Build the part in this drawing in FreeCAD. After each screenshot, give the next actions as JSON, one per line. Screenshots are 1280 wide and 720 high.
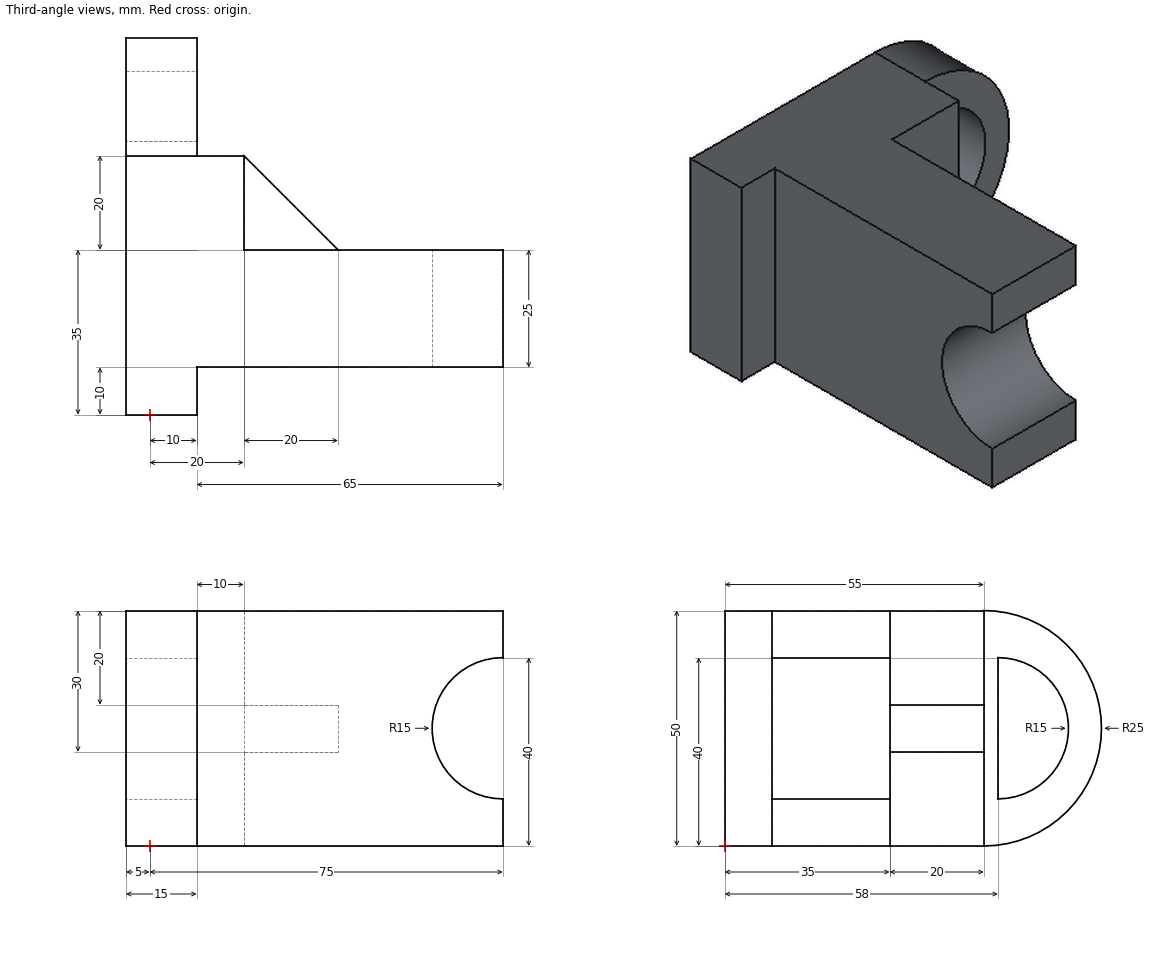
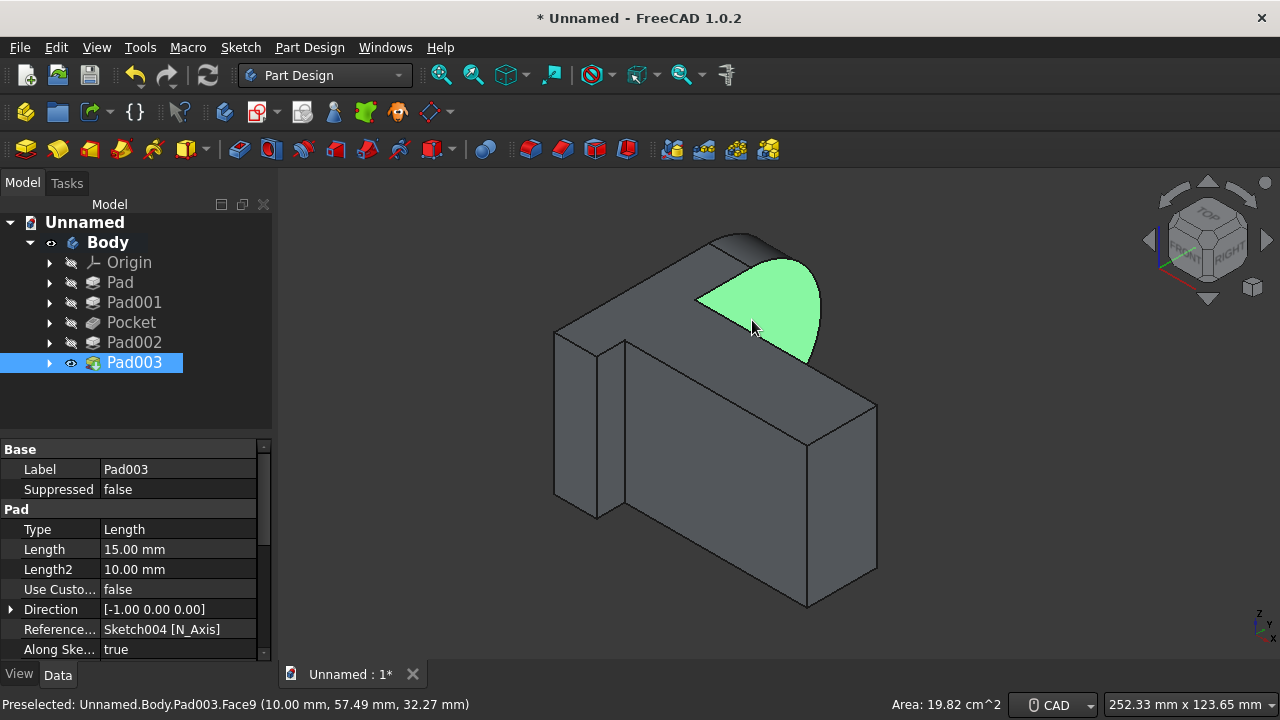
{"action": "left_click", "coordinate": [258, 112]}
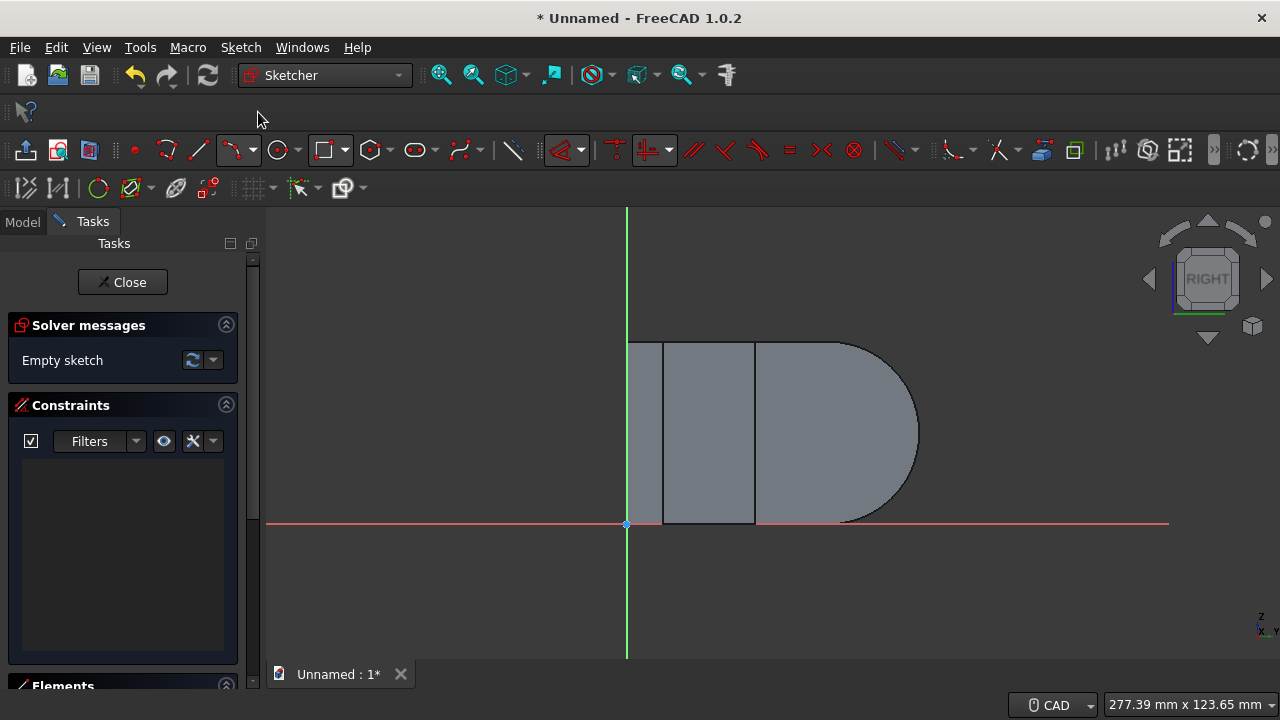
{"action": "scroll", "coordinate": [774, 433], "scroll_direction": "up", "scroll_amount": 2}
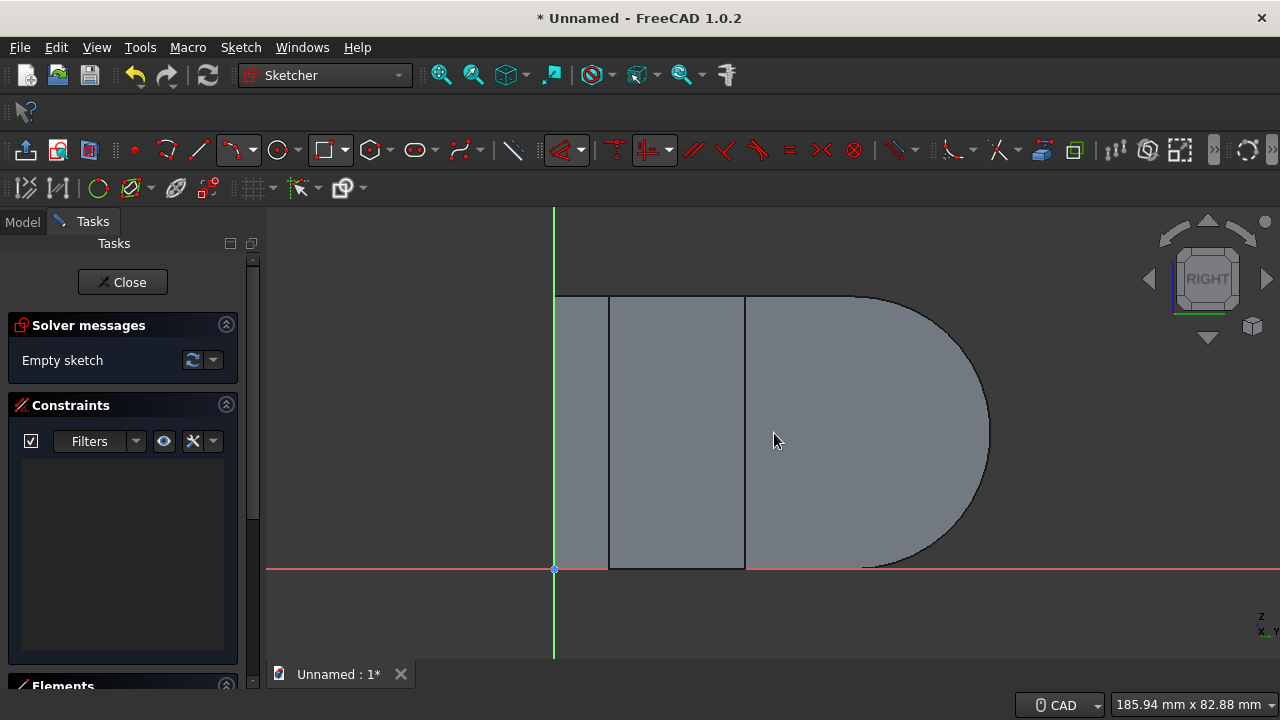
{"action": "key", "text": "g r"}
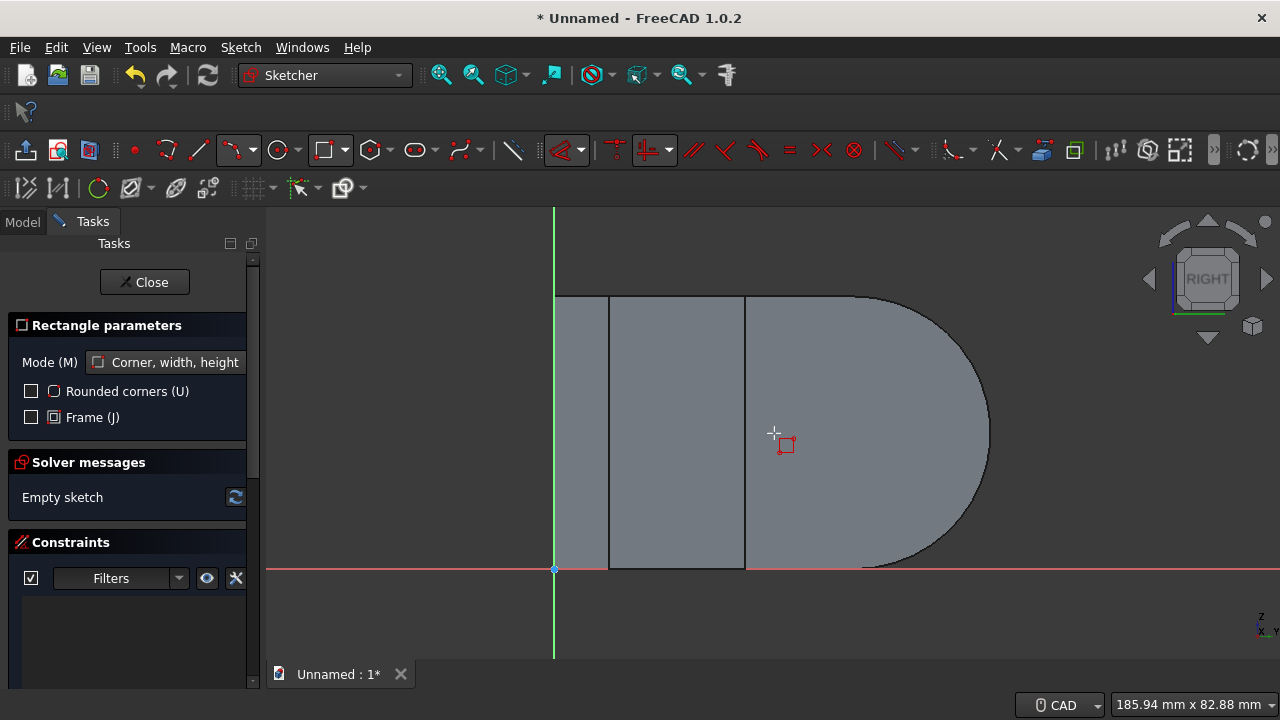
{"action": "left_click", "coordinate": [745, 296]}
{"action": "left_click", "coordinate": [854, 569]}
{"action": "key", "text": "Escape"}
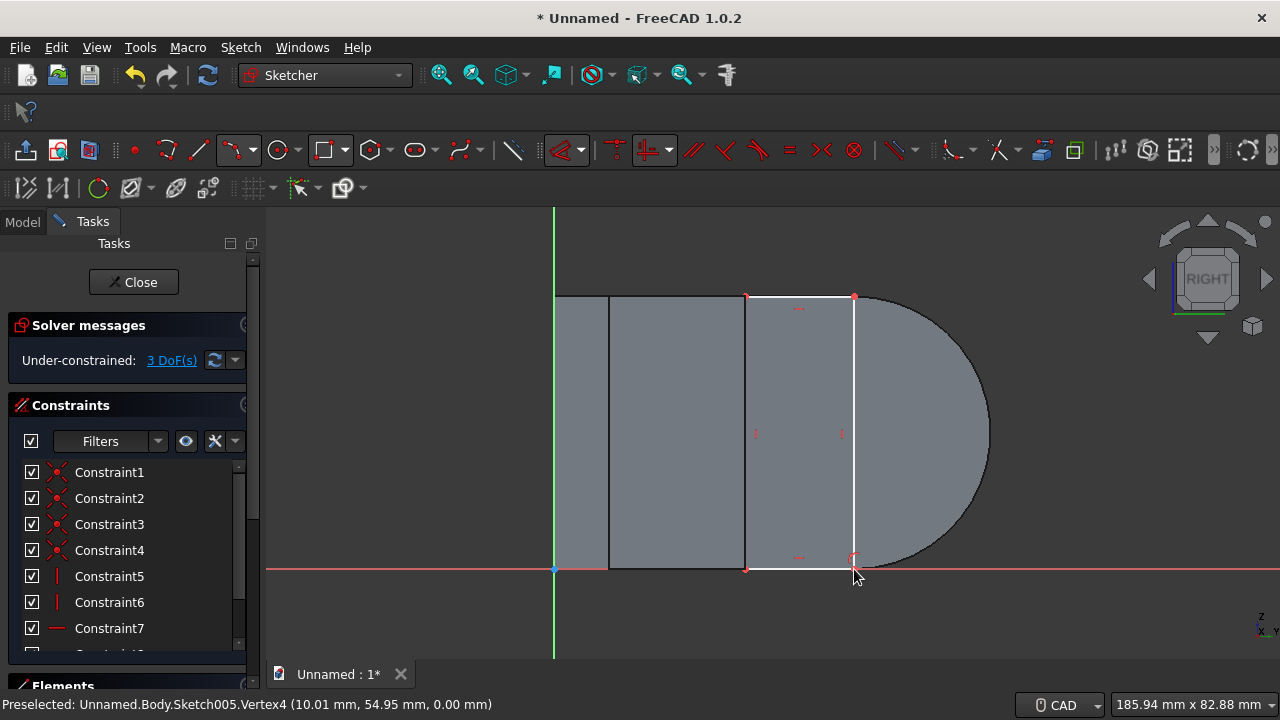
{"action": "left_click", "coordinate": [745, 379]}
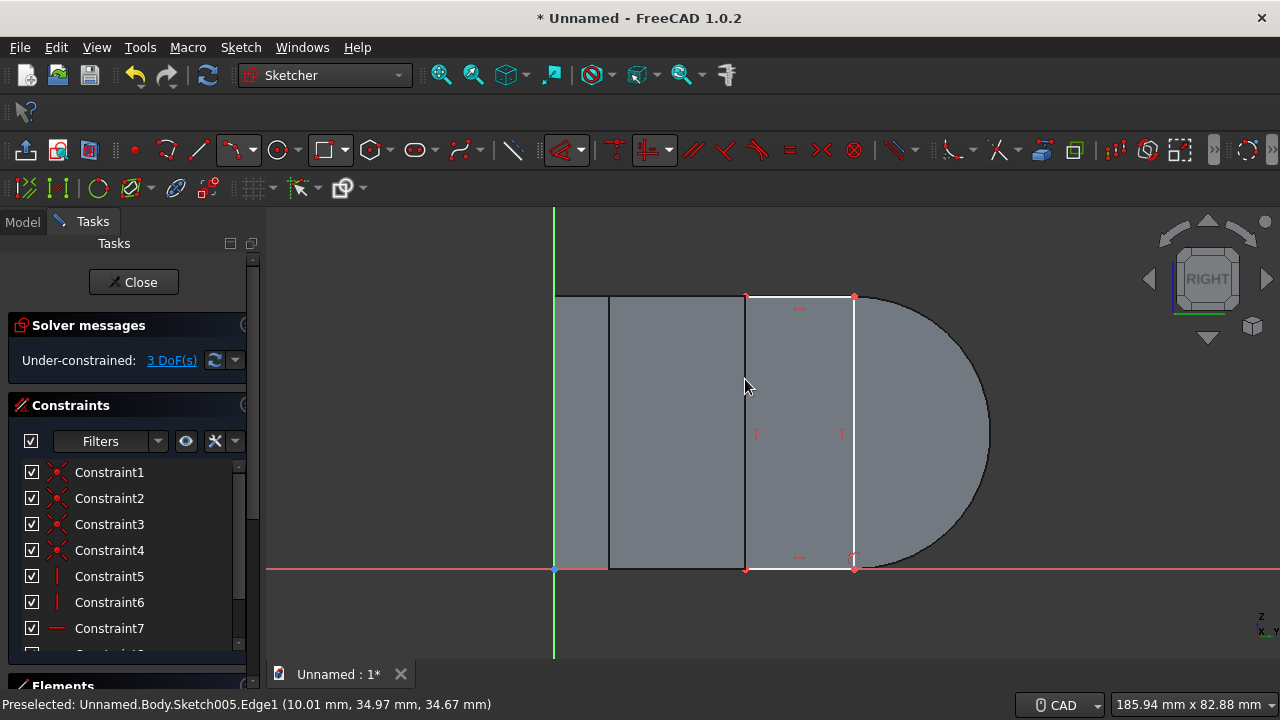
{"action": "left_click", "coordinate": [584, 150]}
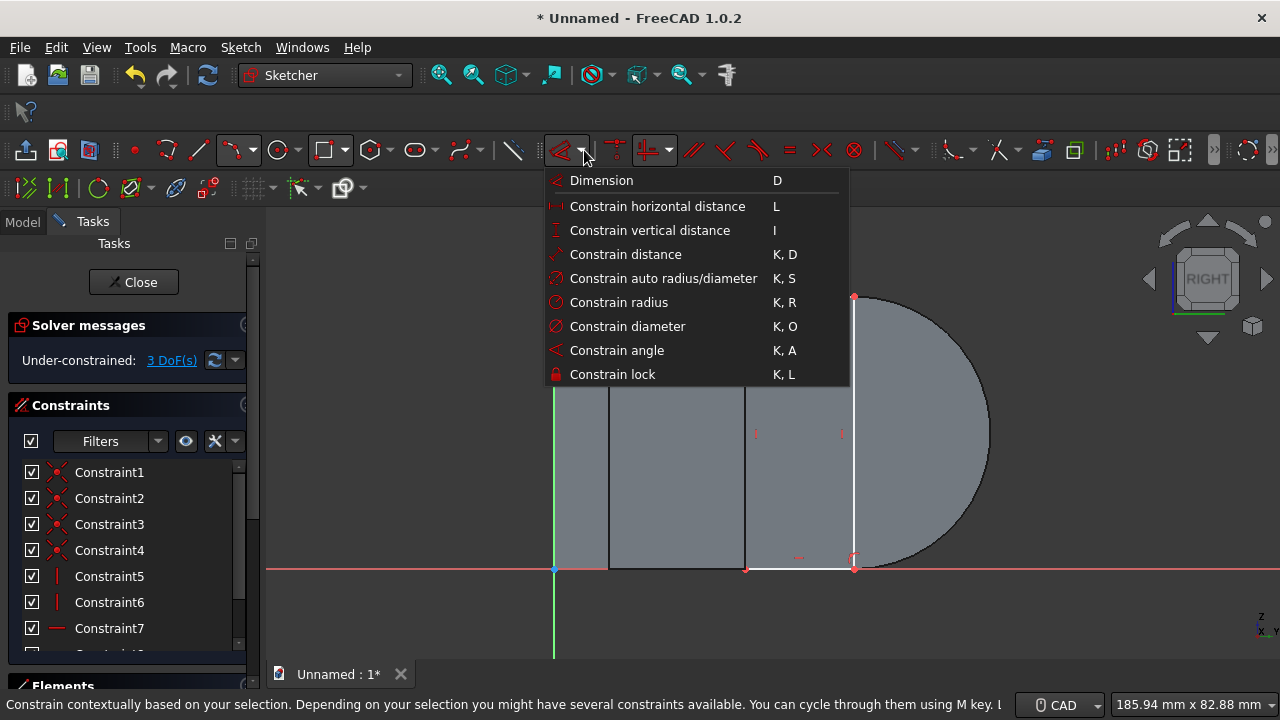
{"action": "left_click", "coordinate": [697, 230]}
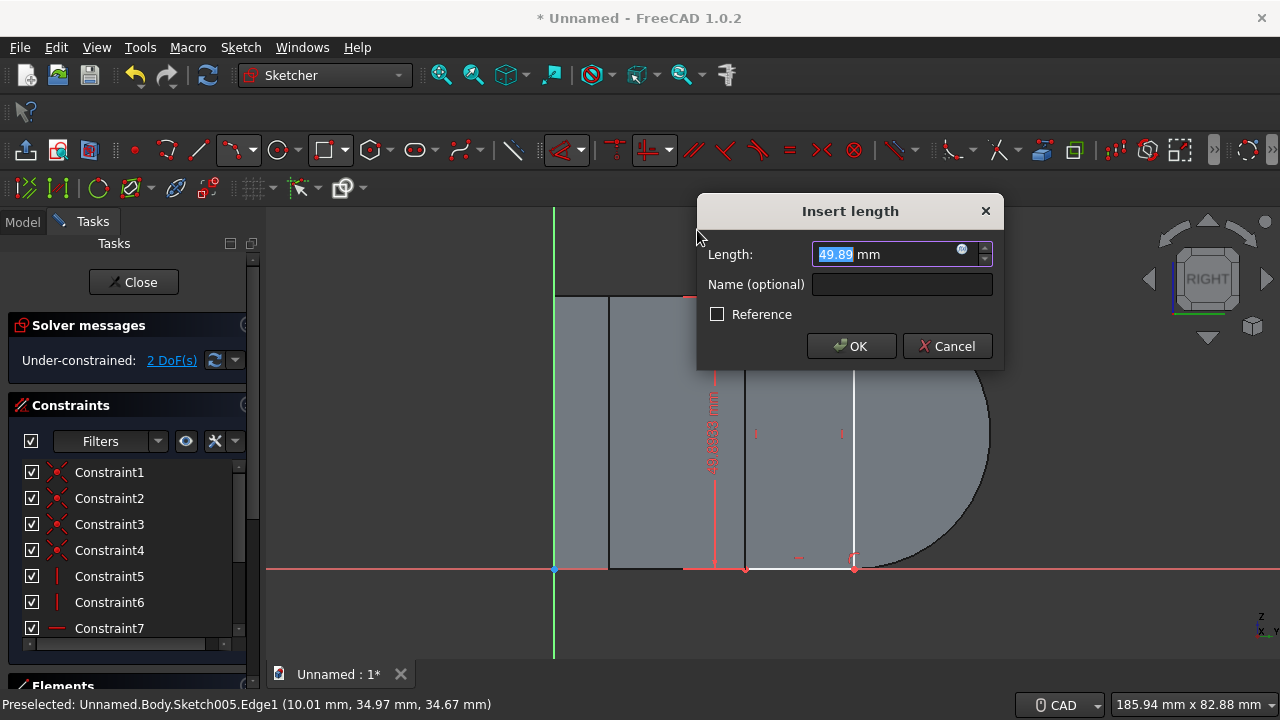
{"action": "type", "text": "50"}
{"action": "key", "text": "Return"}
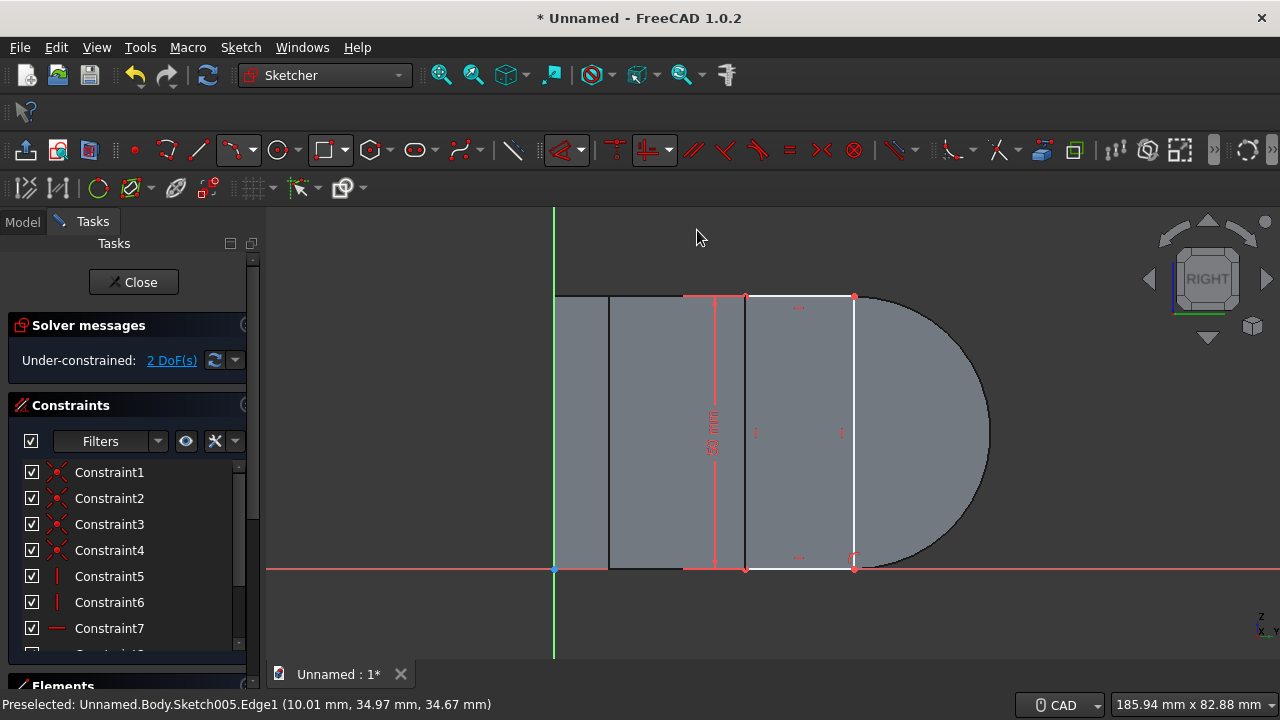
{"action": "left_click", "coordinate": [778, 569]}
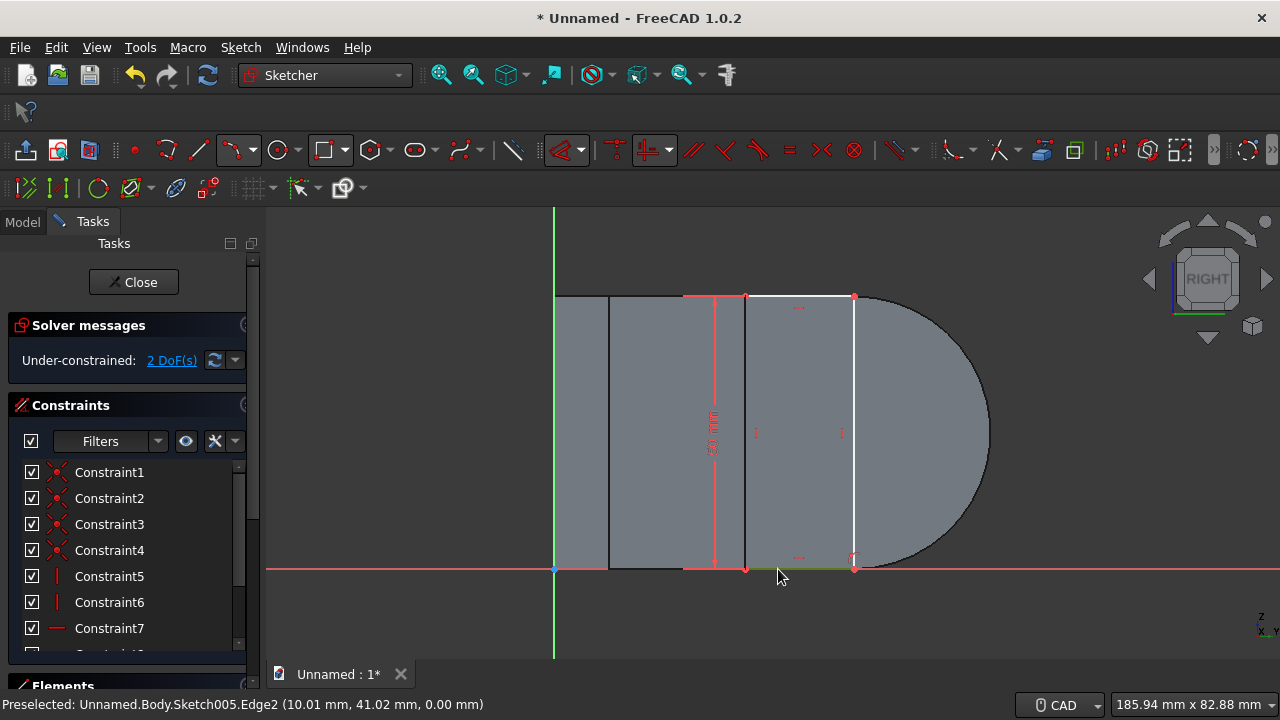
{"action": "key", "text": "l"}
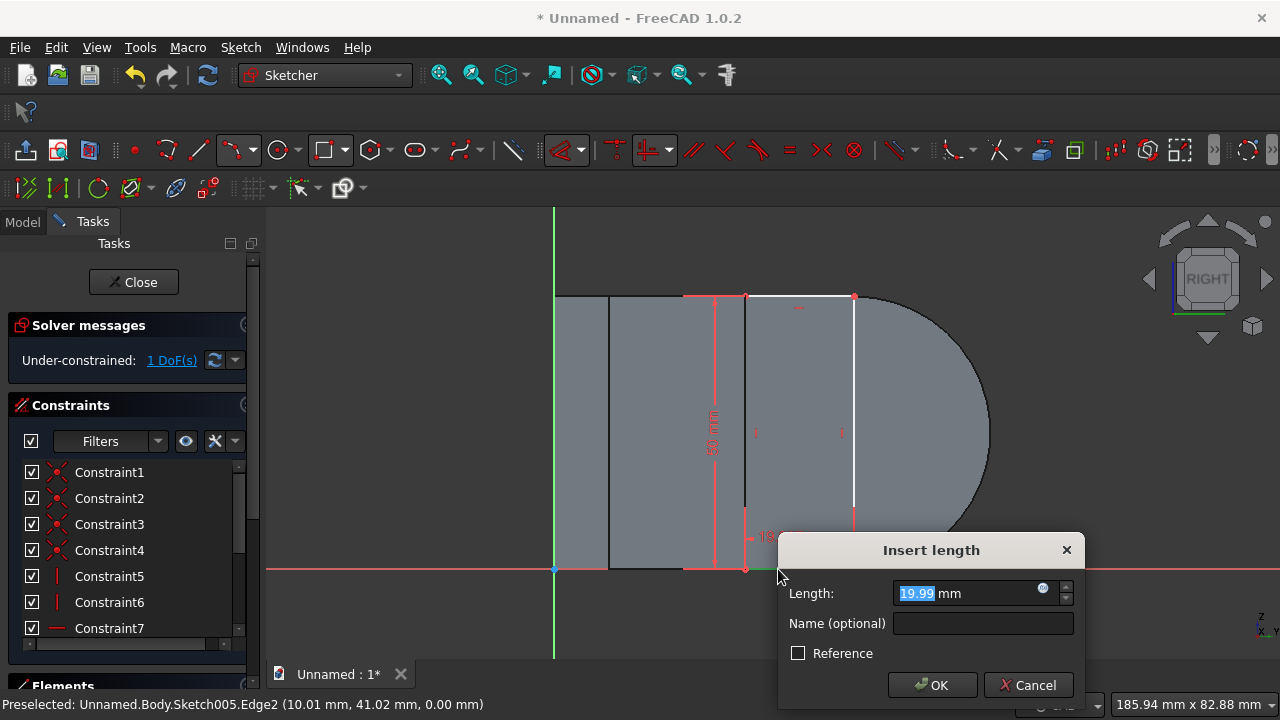
{"action": "type", "text": "20"}
{"action": "key", "text": "Return"}